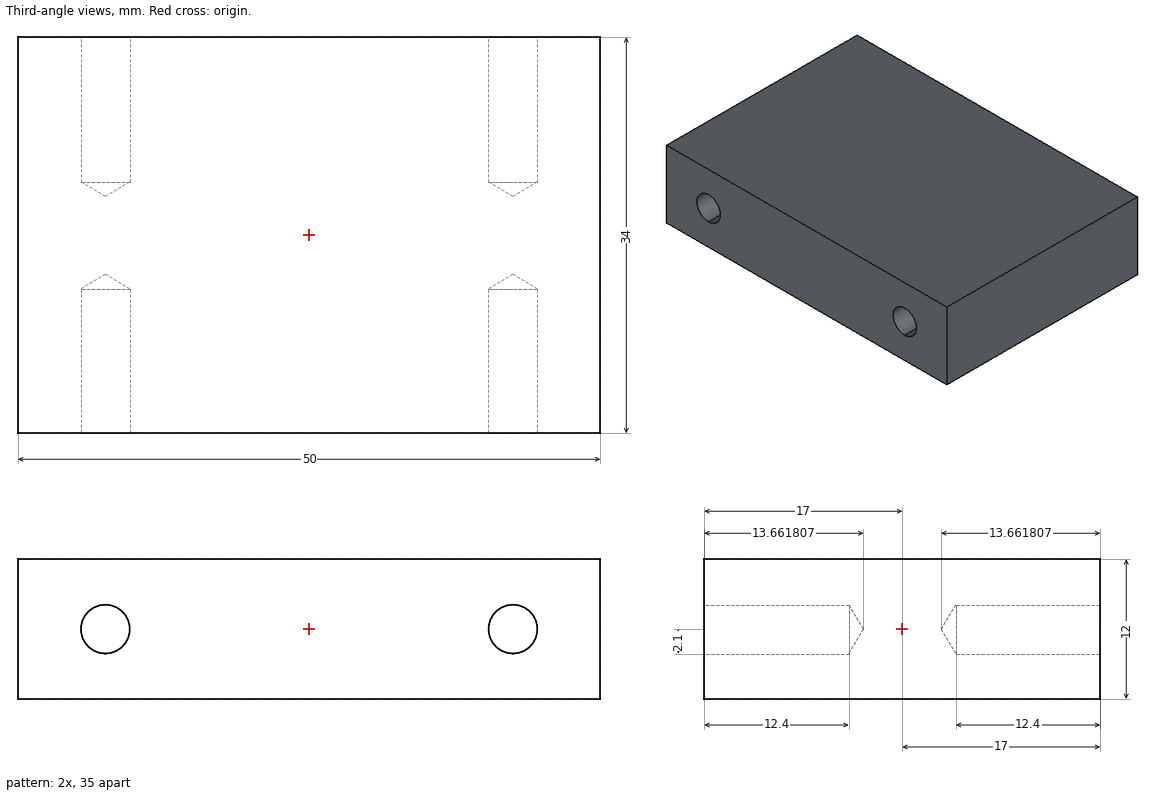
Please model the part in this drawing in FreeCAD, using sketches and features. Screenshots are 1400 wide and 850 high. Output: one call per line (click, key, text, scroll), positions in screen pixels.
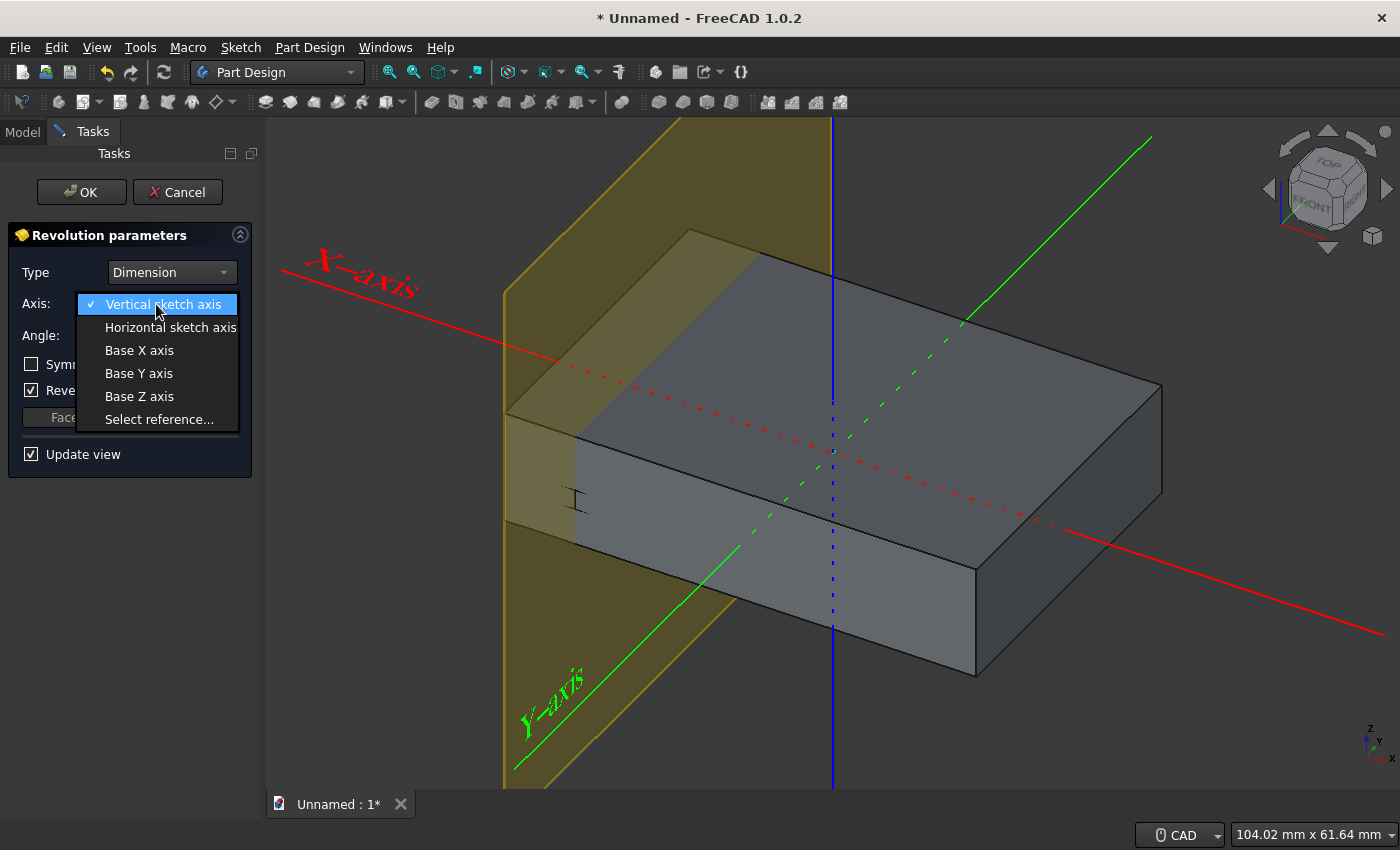
click(156, 328)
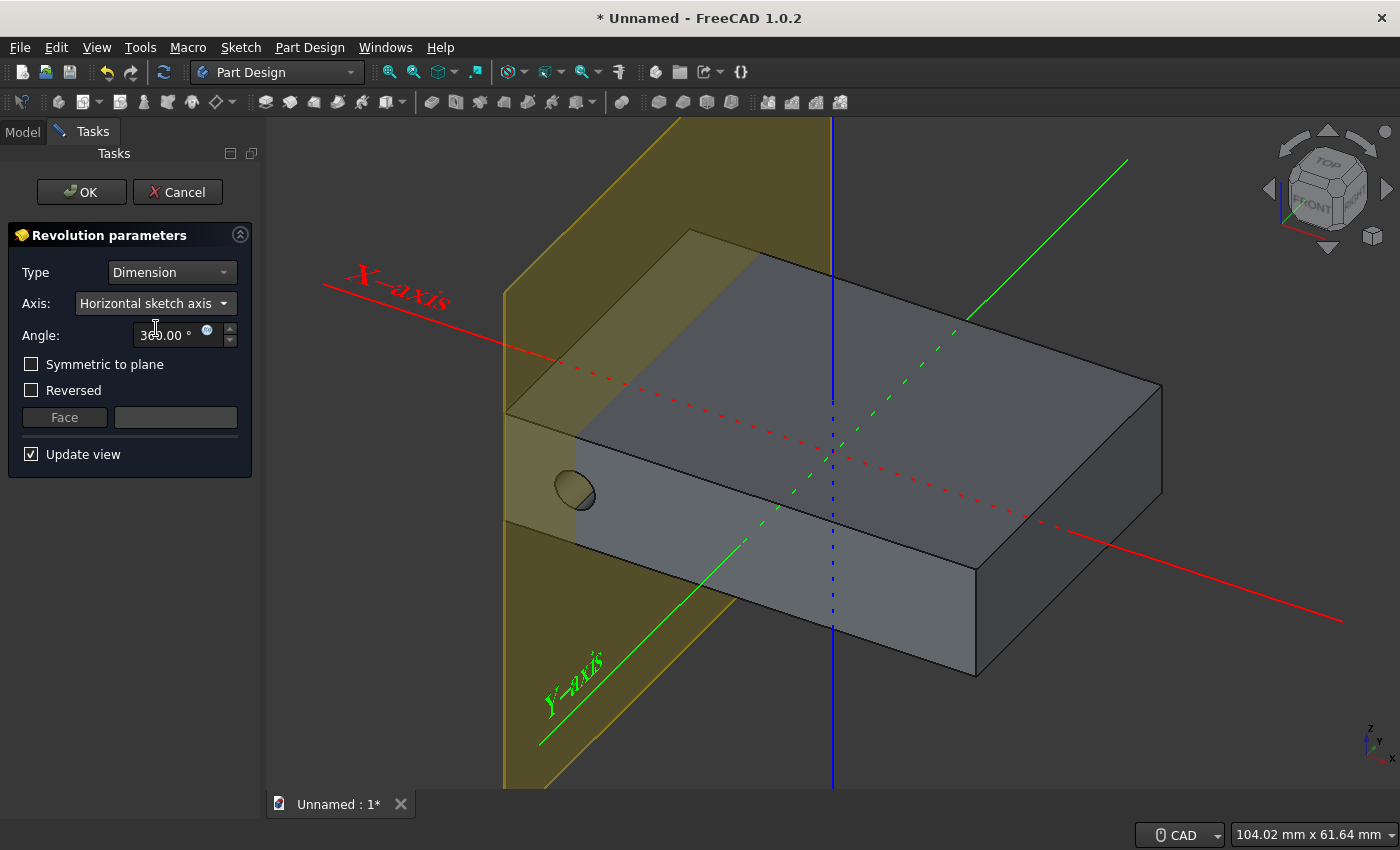
click(82, 192)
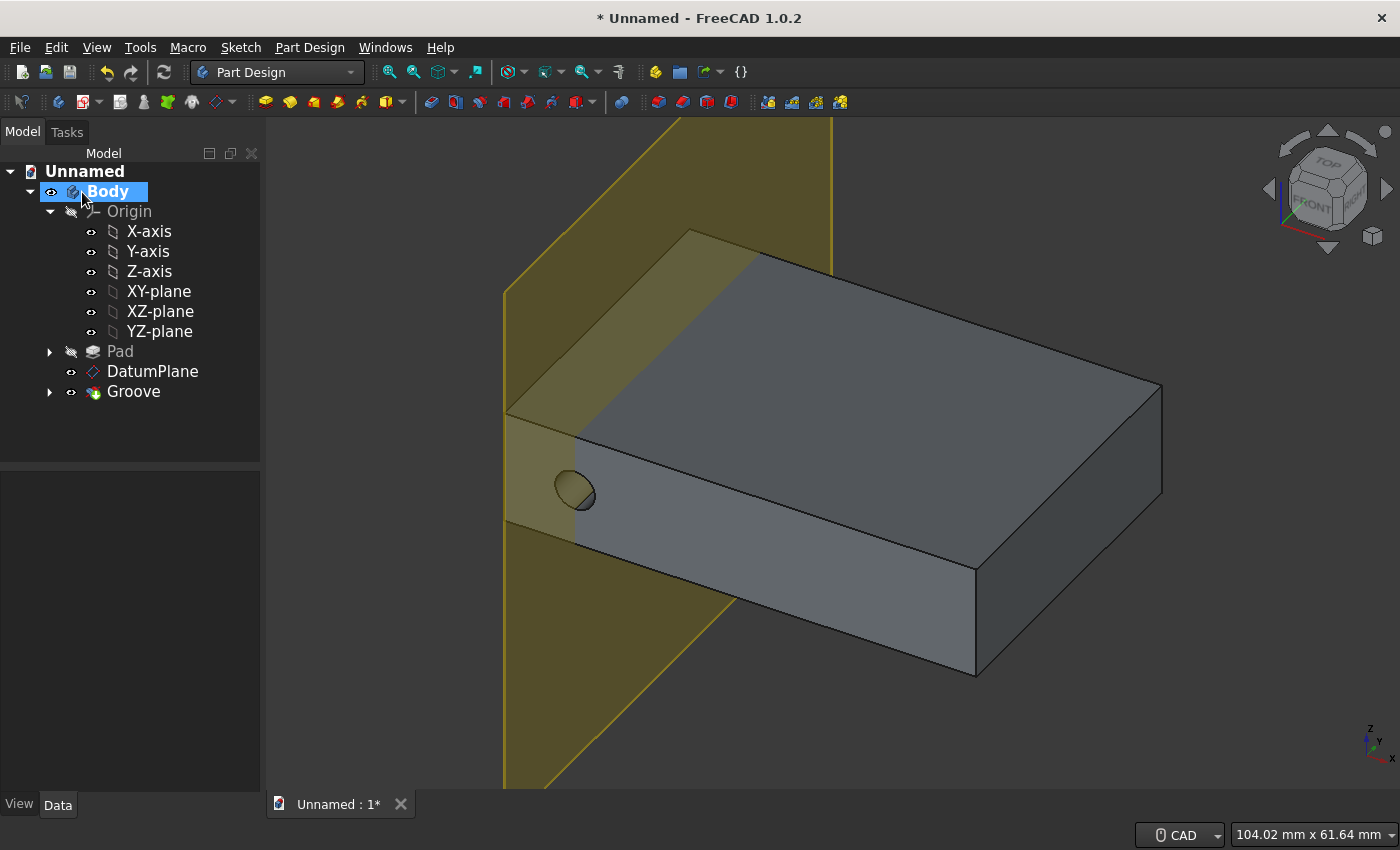
click(116, 372)
key(space)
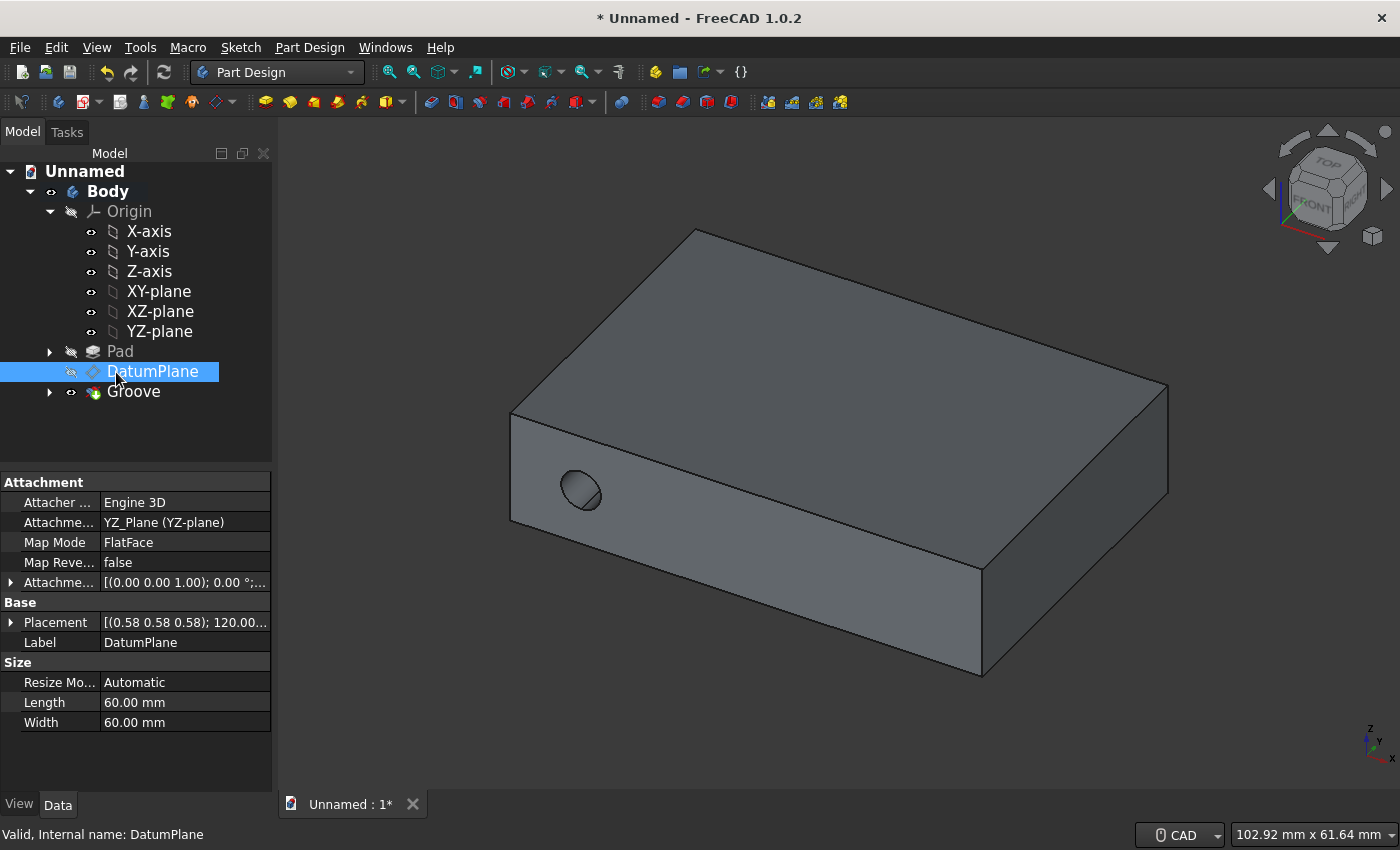
click(116, 392)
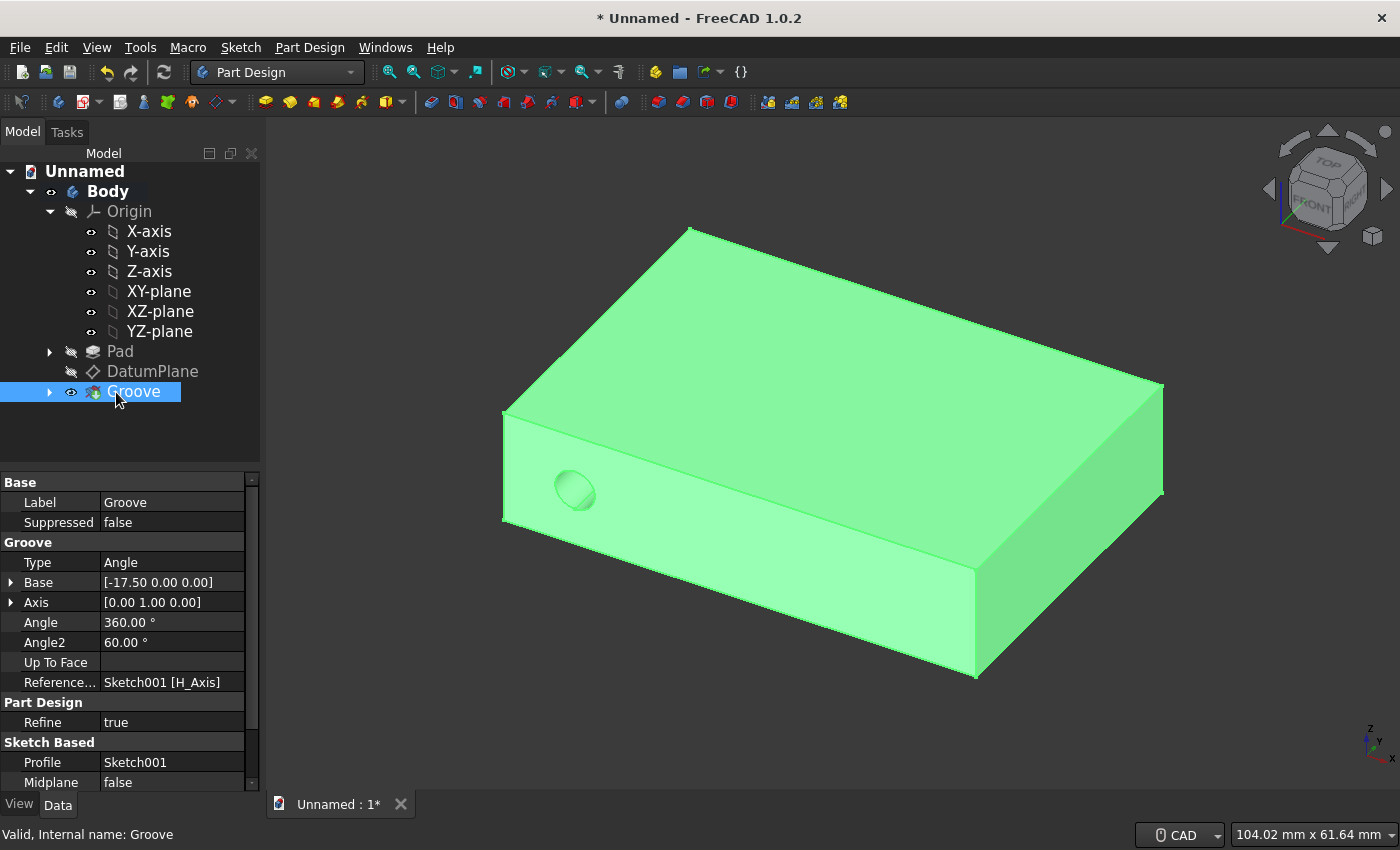
click(792, 102)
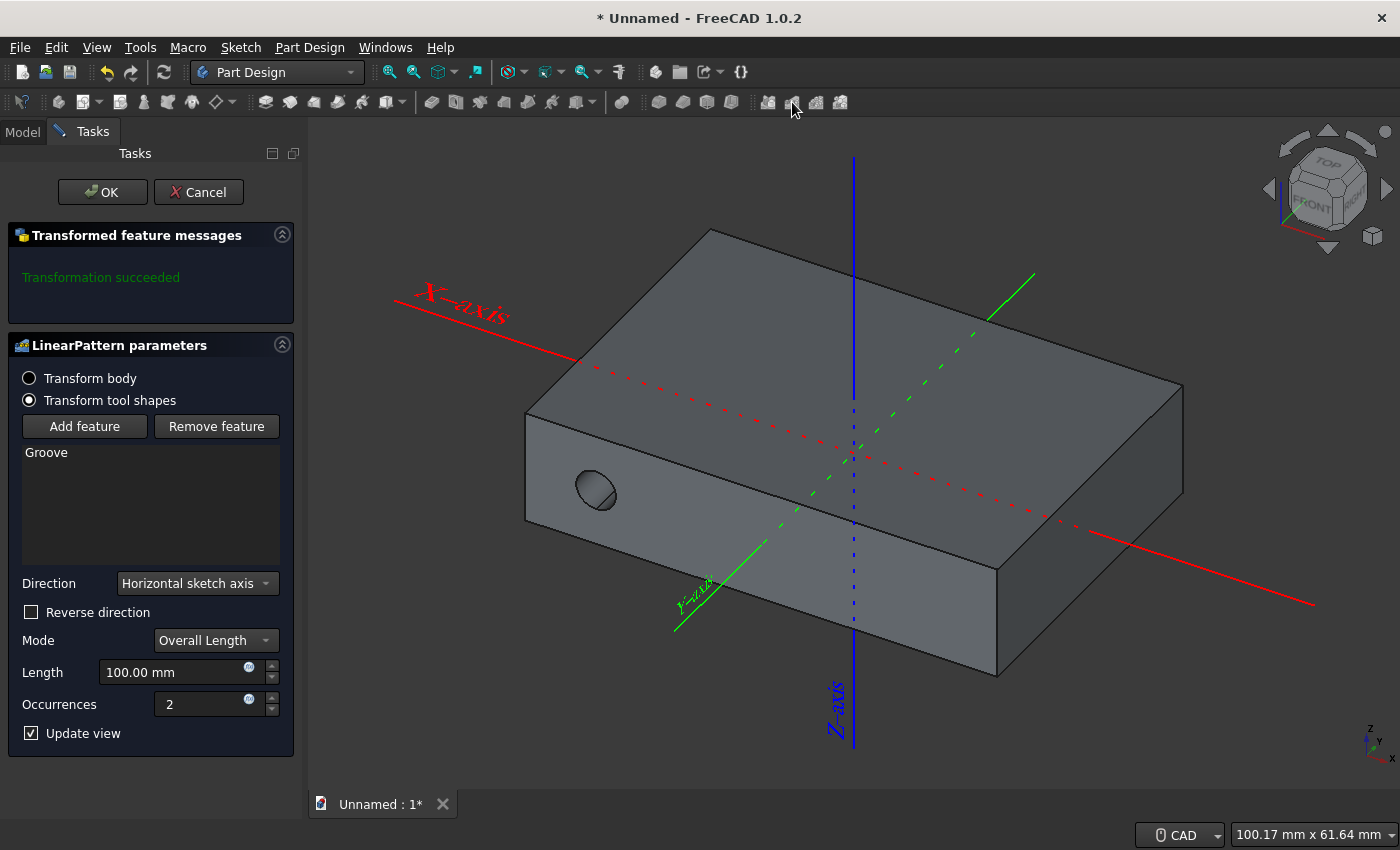
click(198, 584)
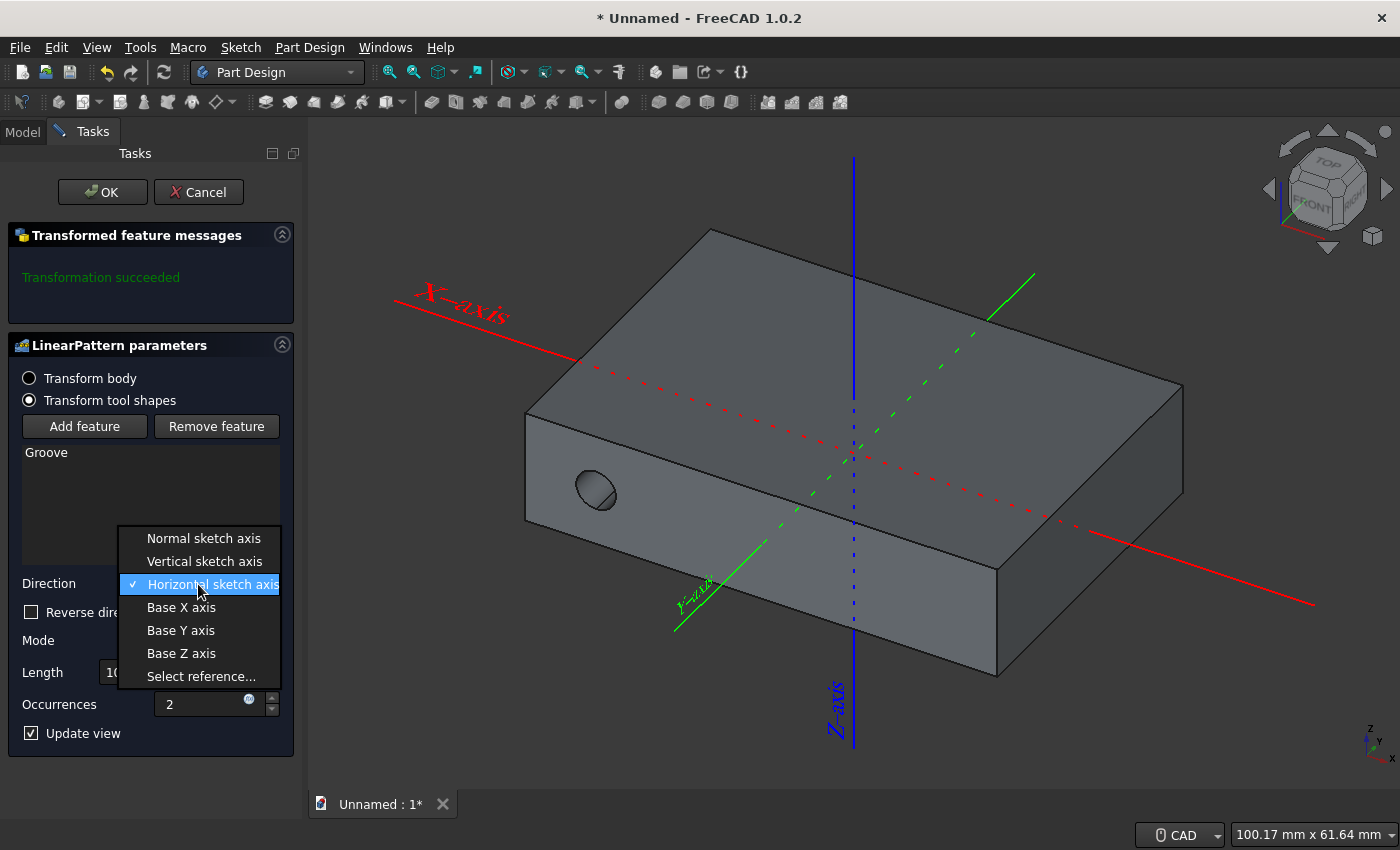
click(198, 608)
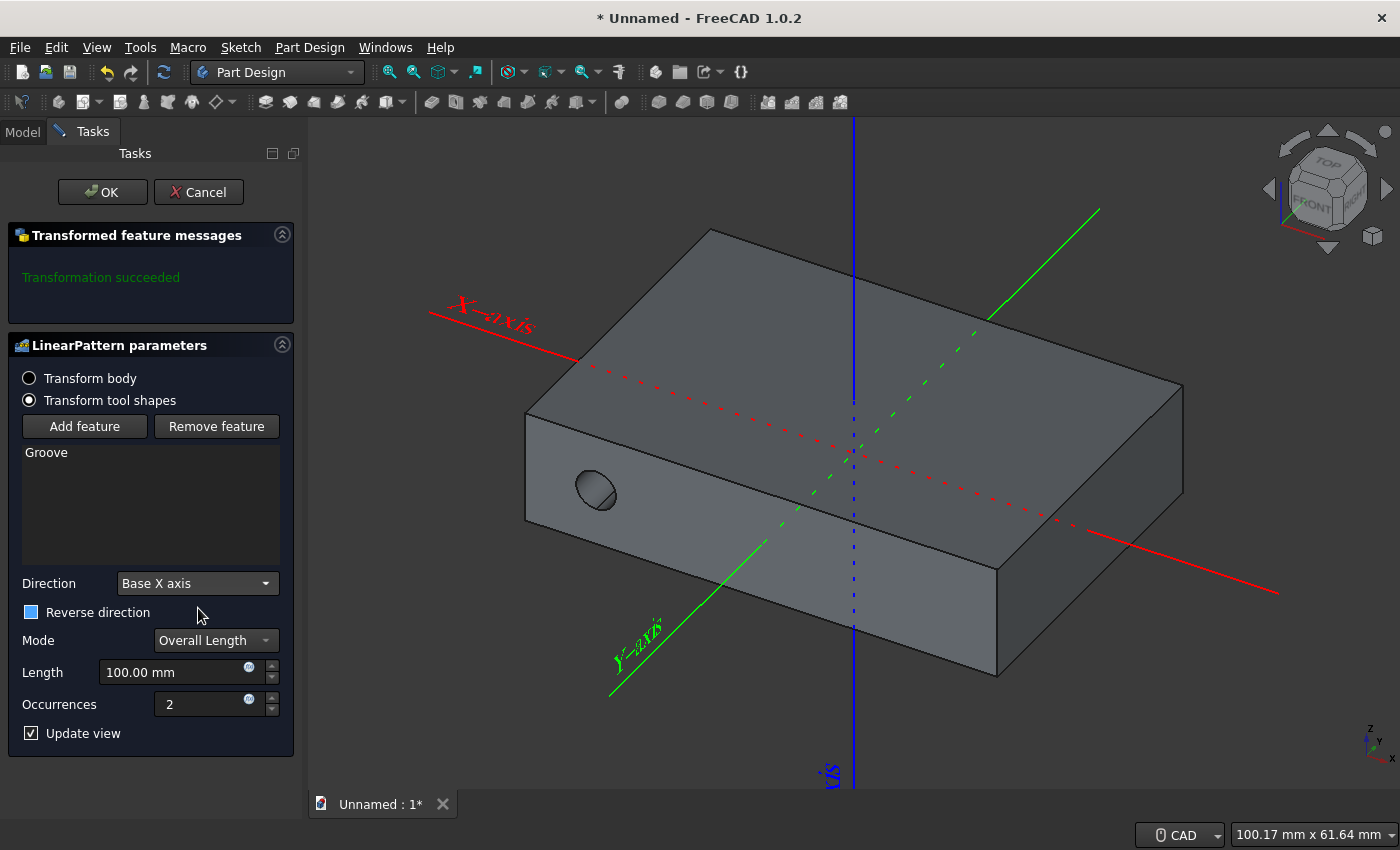
click(217, 640)